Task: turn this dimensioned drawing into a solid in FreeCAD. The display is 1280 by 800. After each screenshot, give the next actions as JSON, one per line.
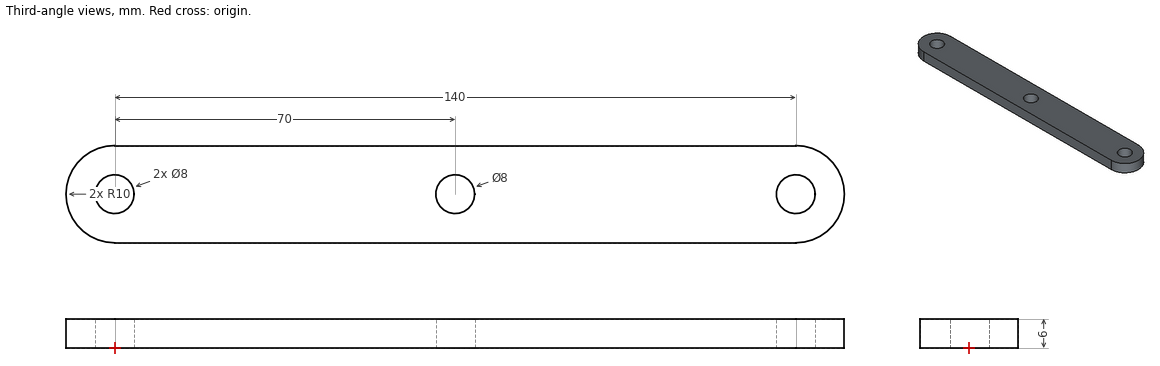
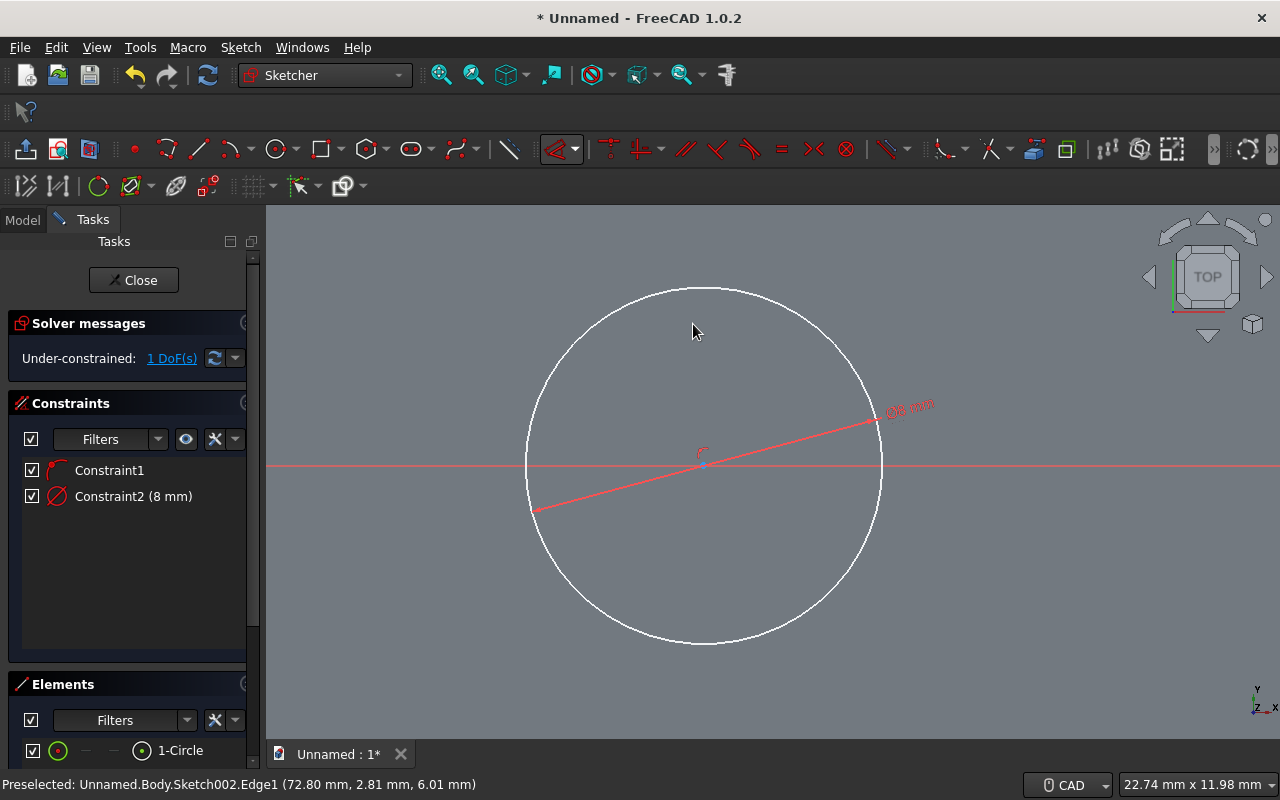
{"action": "left_click", "coordinate": [704, 466]}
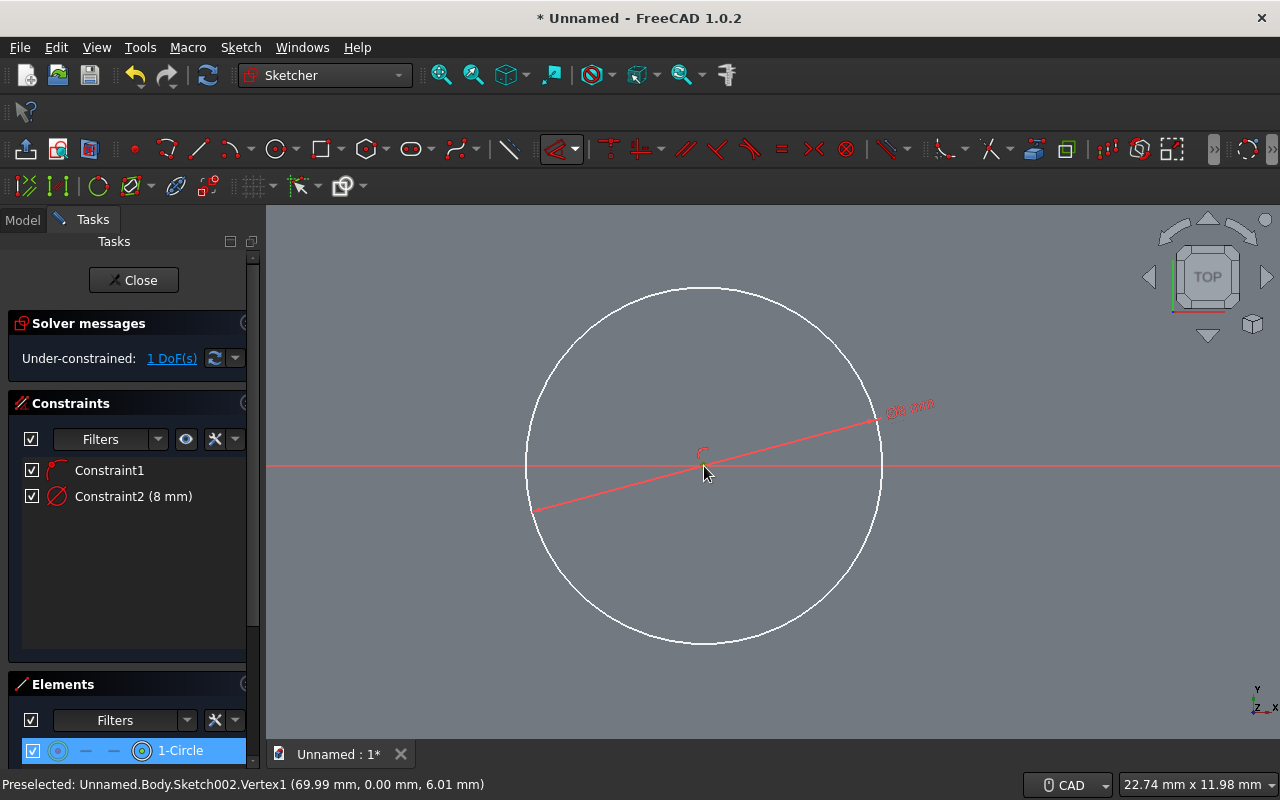
{"action": "key", "text": "l"}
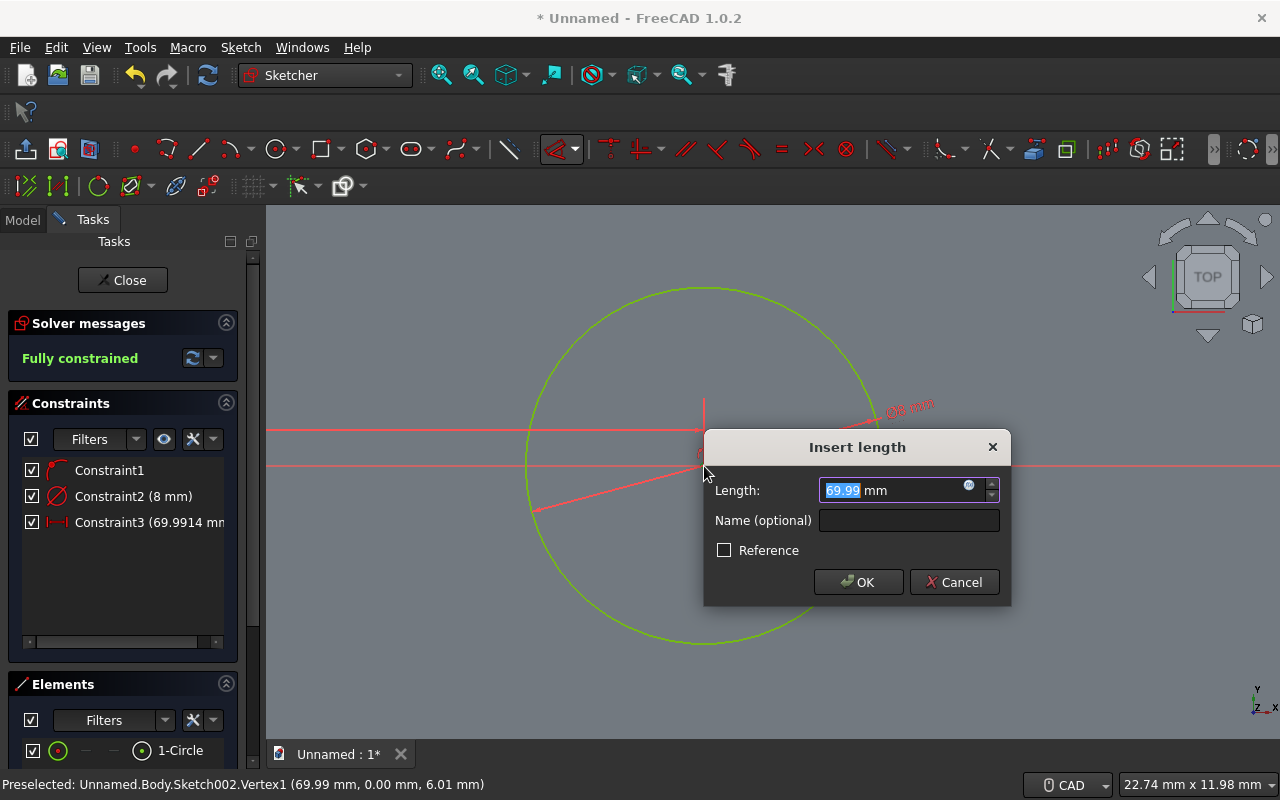
{"action": "type", "text": "70"}
{"action": "key", "text": "Return"}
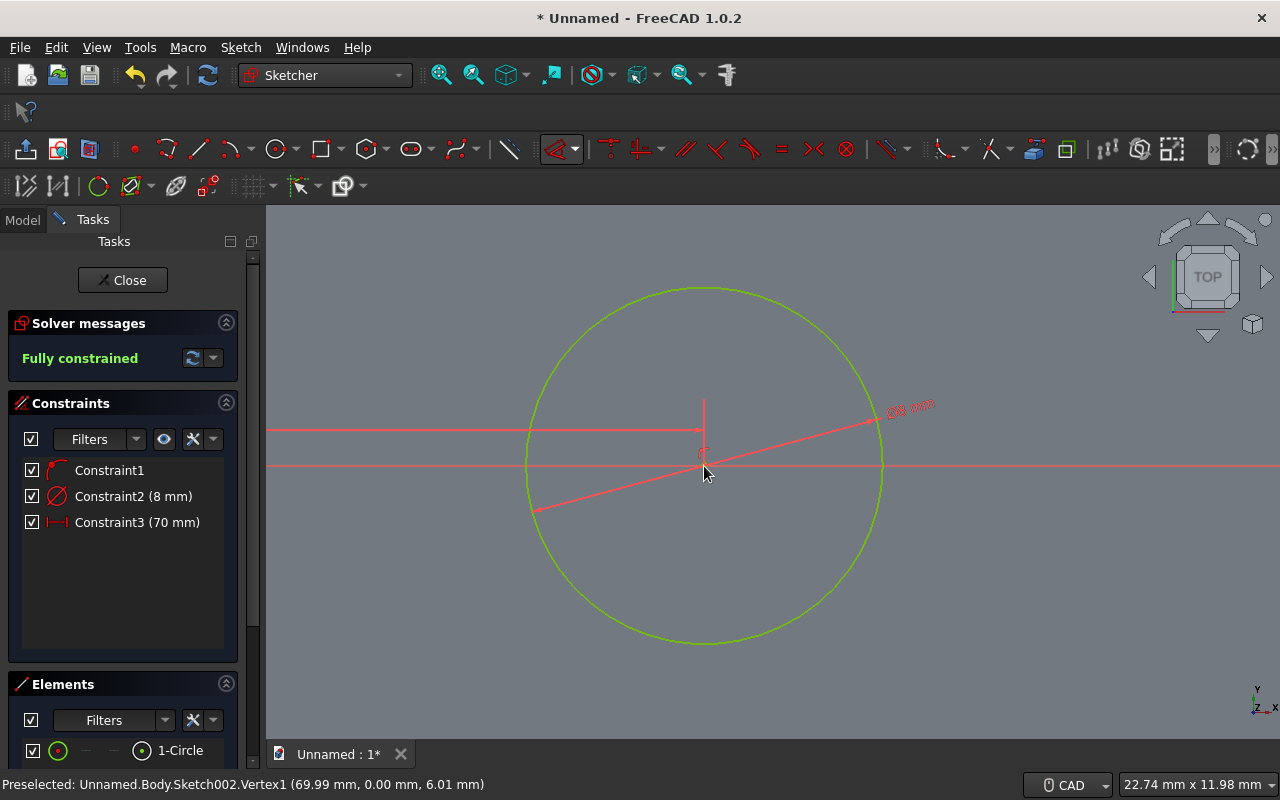
{"action": "left_click", "coordinate": [123, 280]}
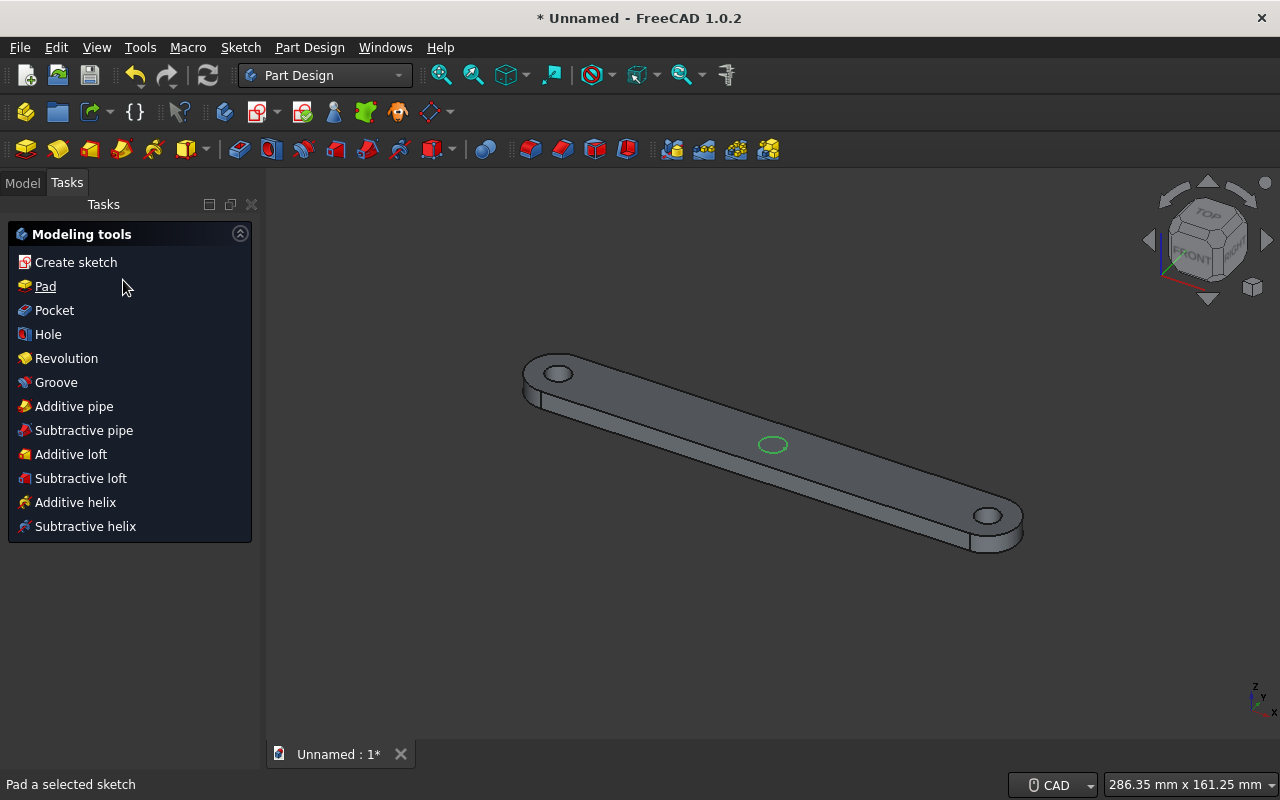
{"action": "left_click", "coordinate": [240, 150]}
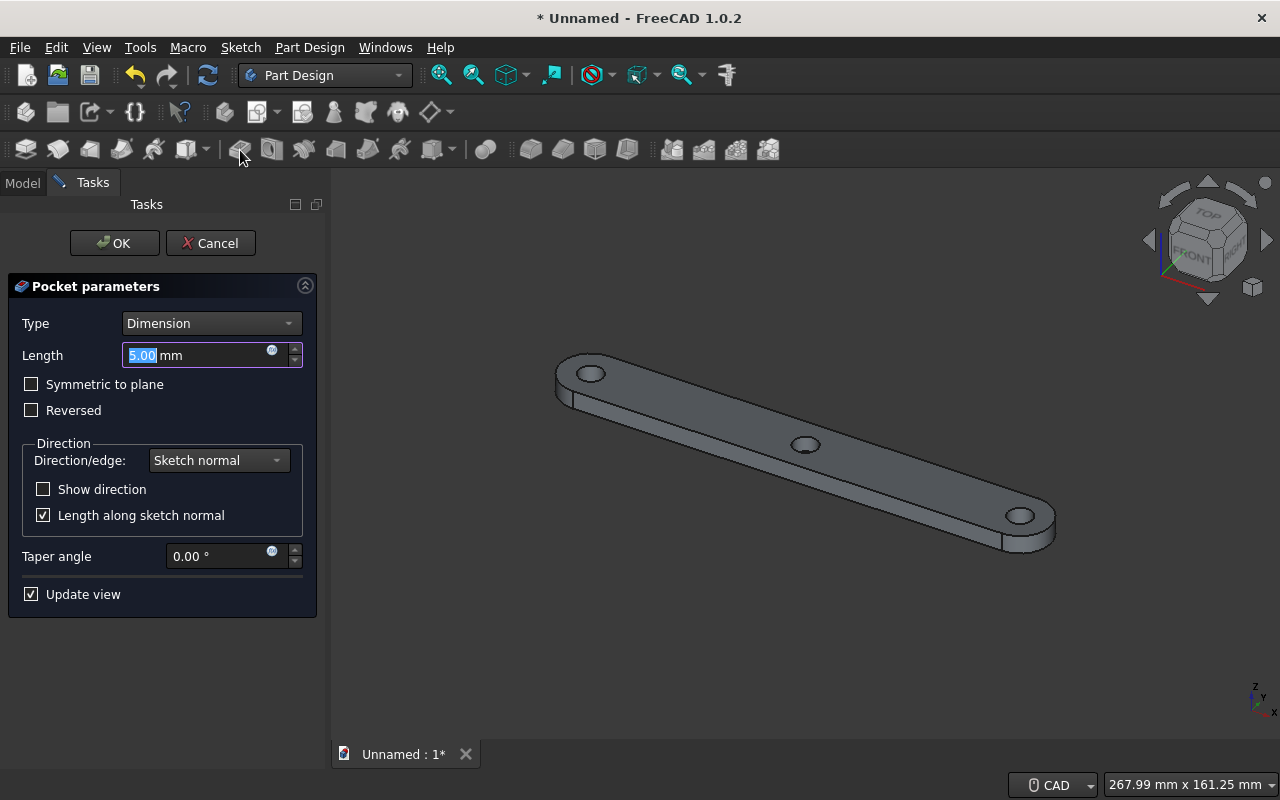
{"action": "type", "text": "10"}
{"action": "key", "text": "Tab"}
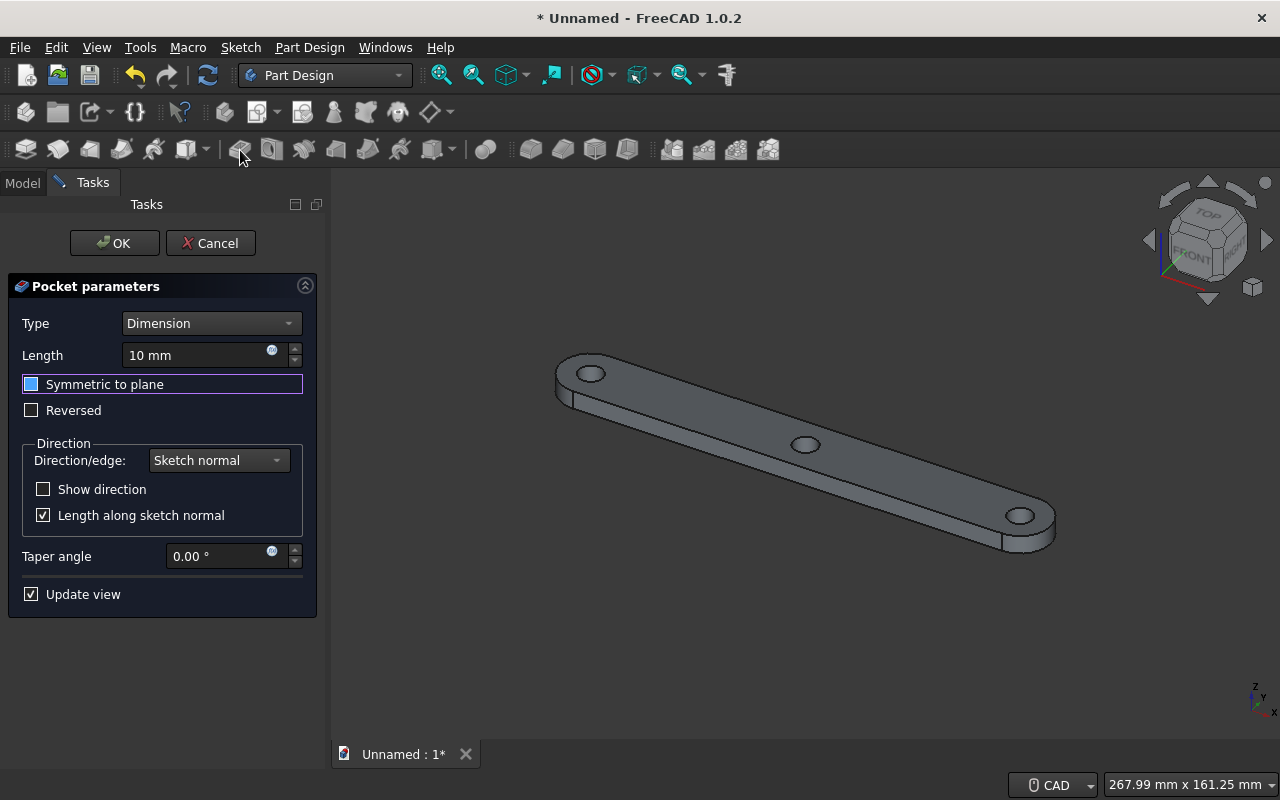
{"action": "left_click", "coordinate": [115, 243]}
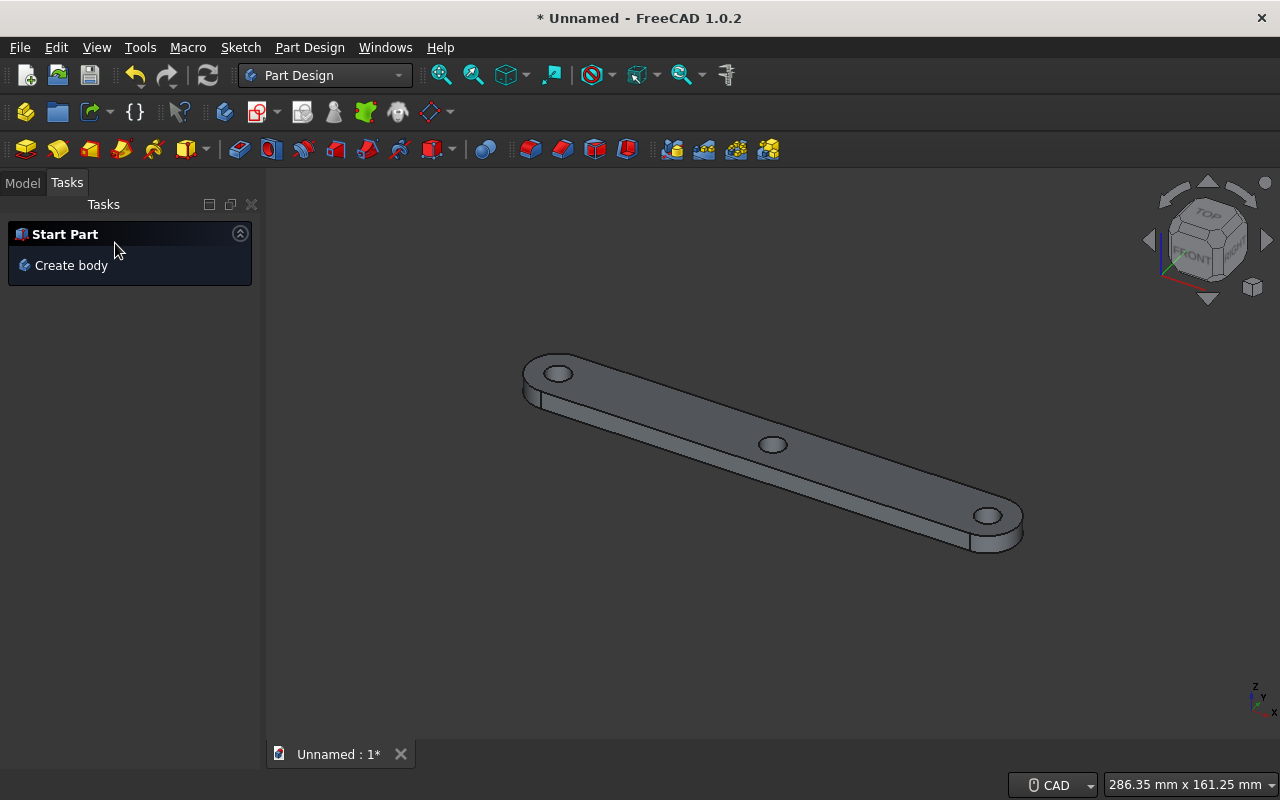
{"action": "key", "text": "0"}